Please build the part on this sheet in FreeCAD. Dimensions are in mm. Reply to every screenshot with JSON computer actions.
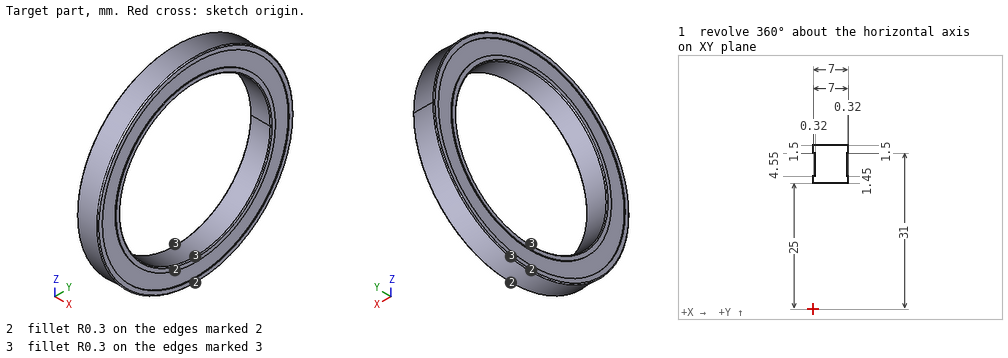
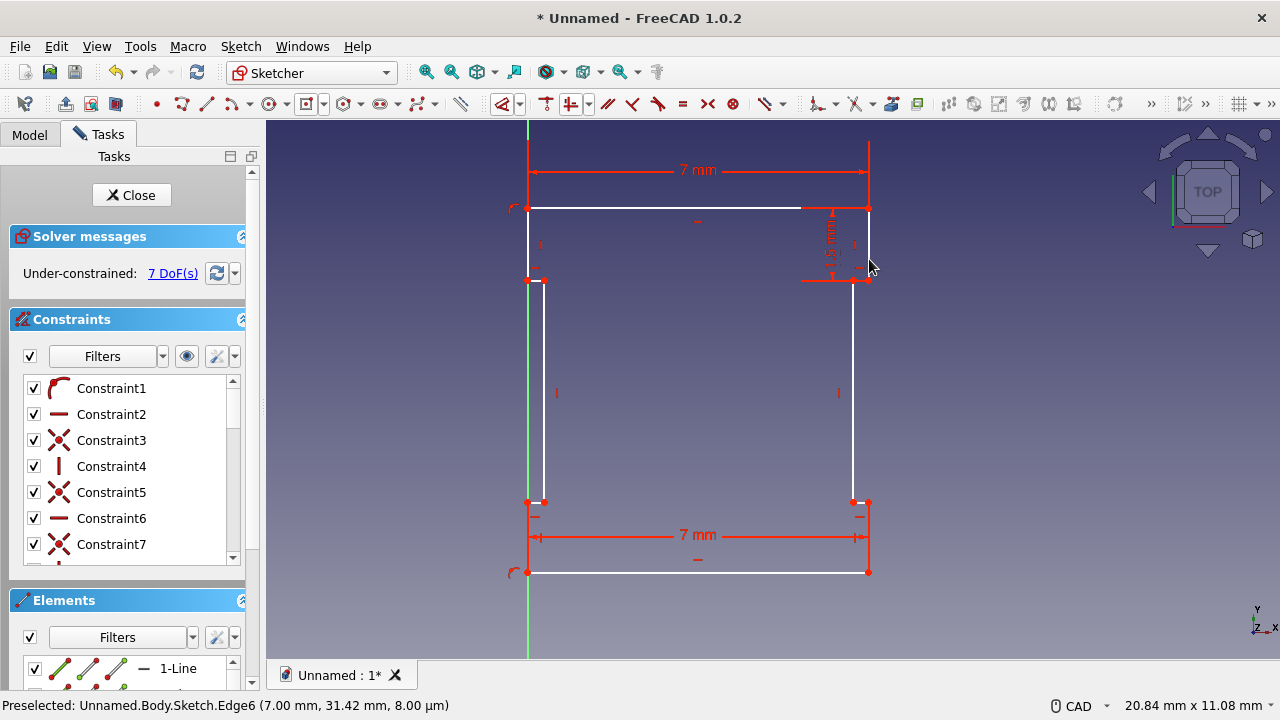
{"action": "left_click", "coordinate": [528, 230]}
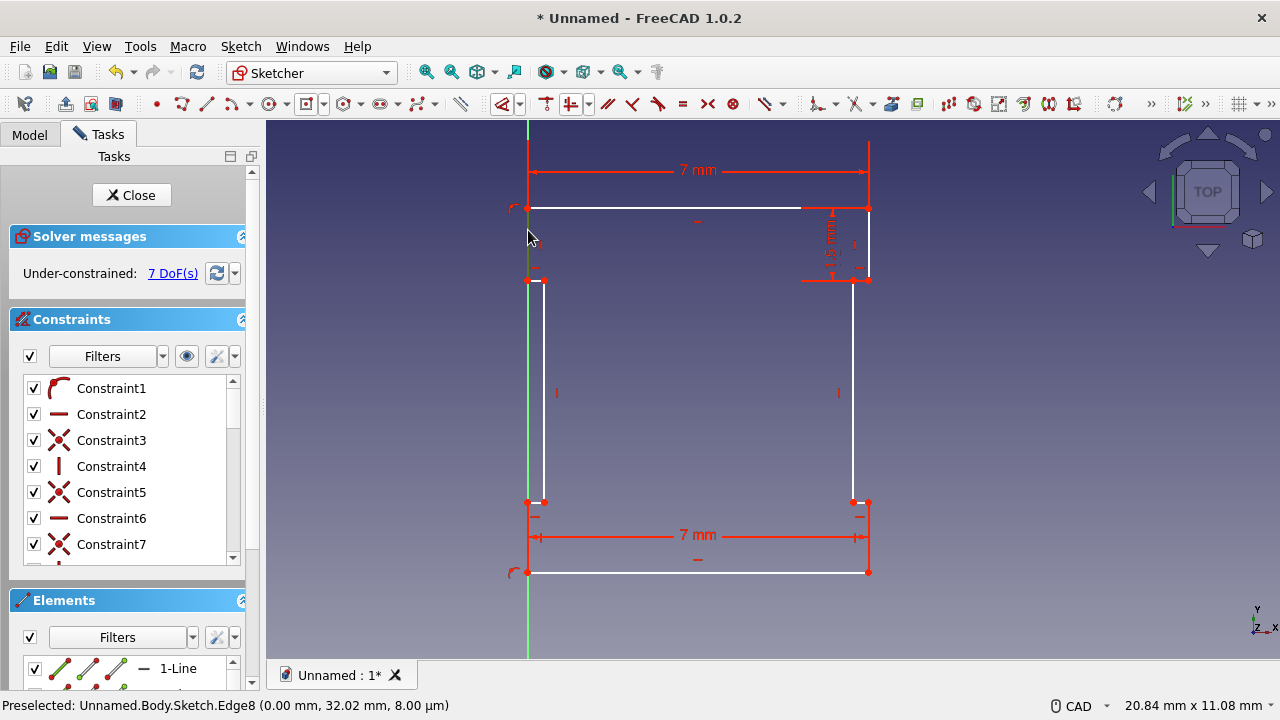
{"action": "left_click", "coordinate": [520, 104]}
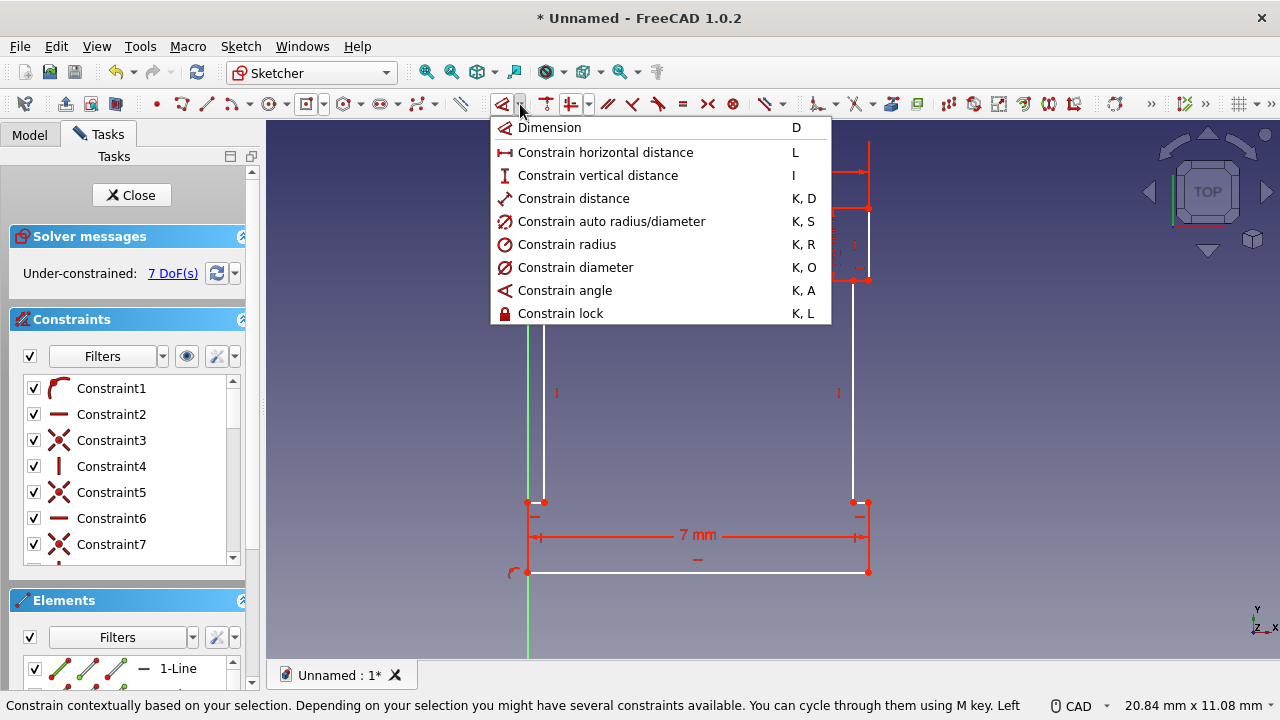
{"action": "left_click", "coordinate": [661, 176]}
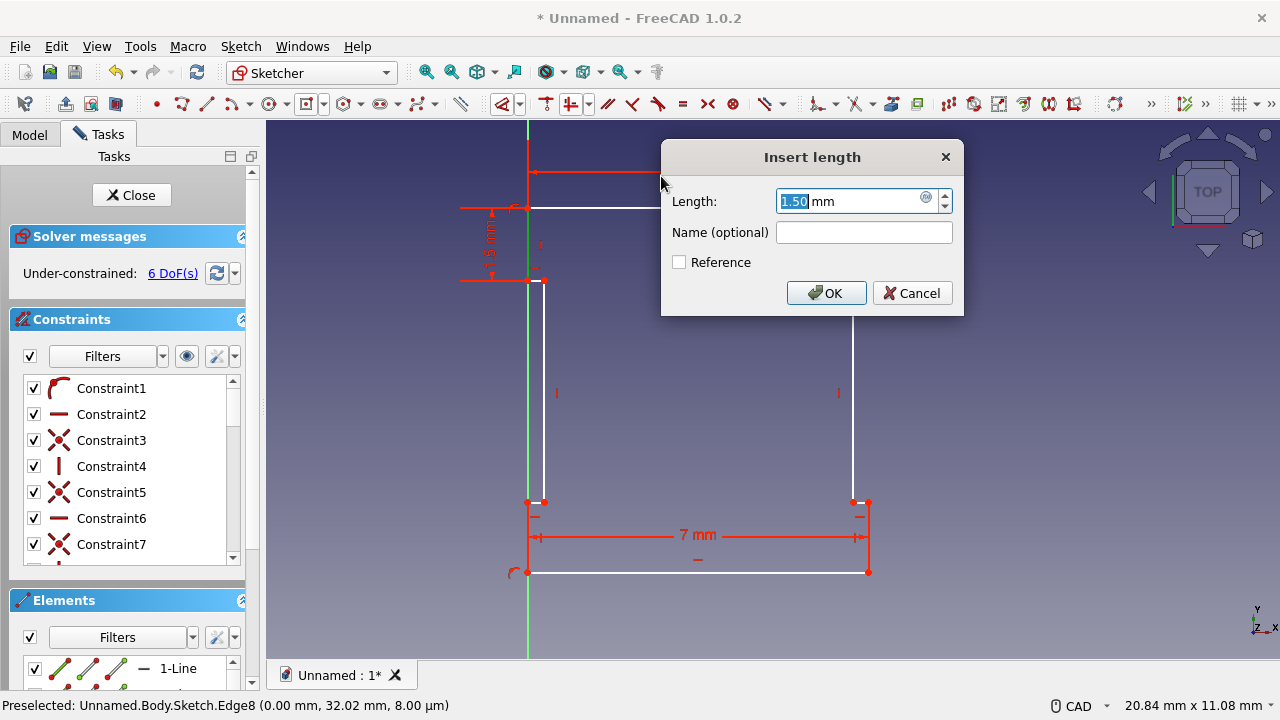
{"action": "type", "text": "1.5"}
{"action": "key", "text": "Return"}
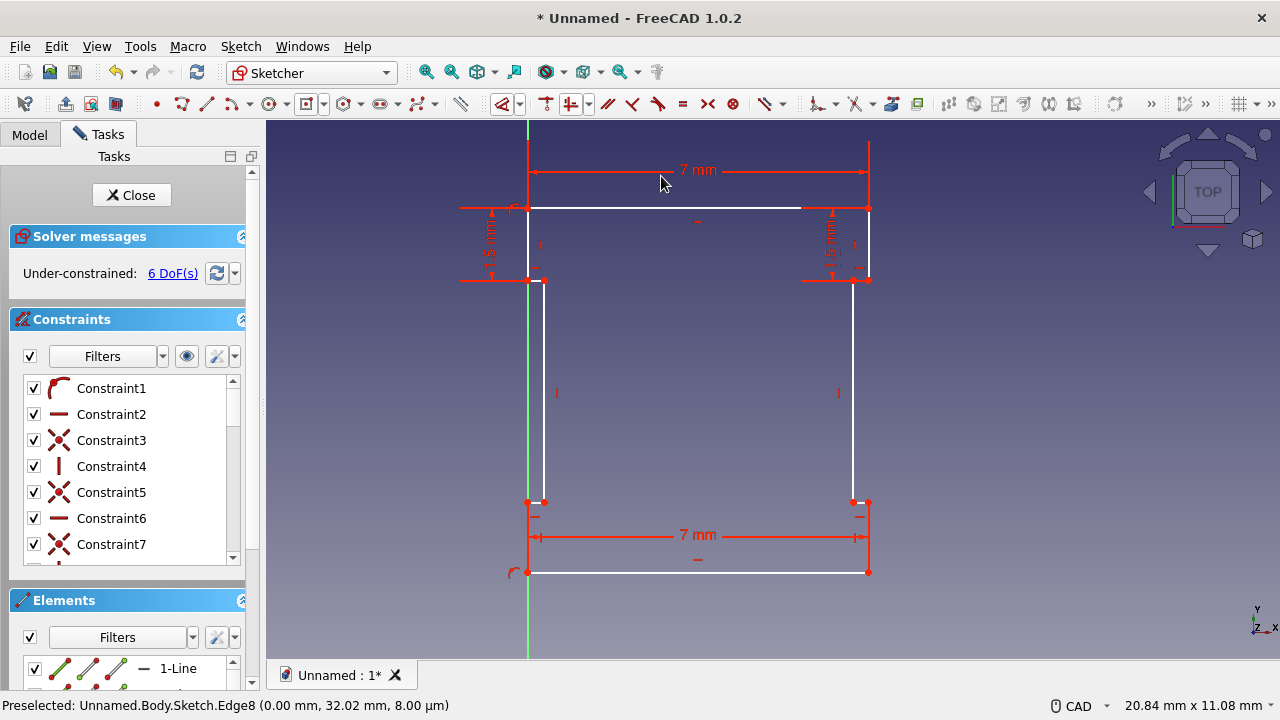
{"action": "left_click", "coordinate": [528, 573]}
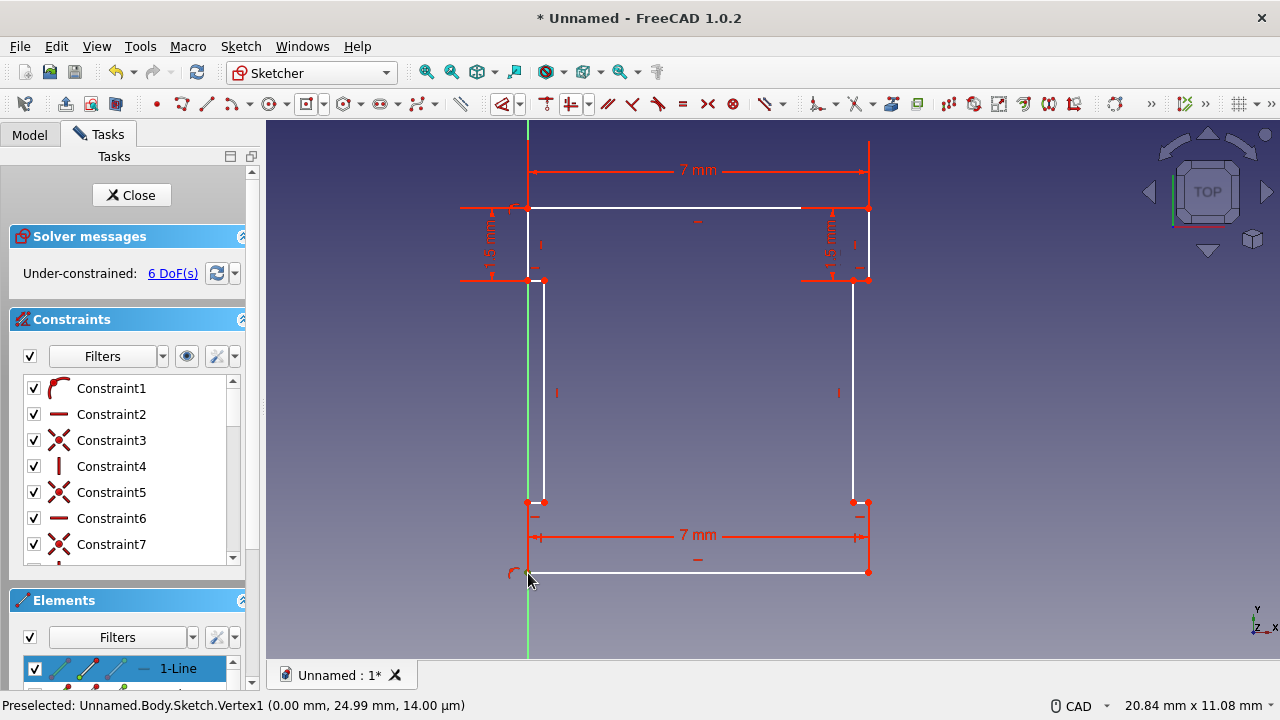
{"action": "key", "text": "i"}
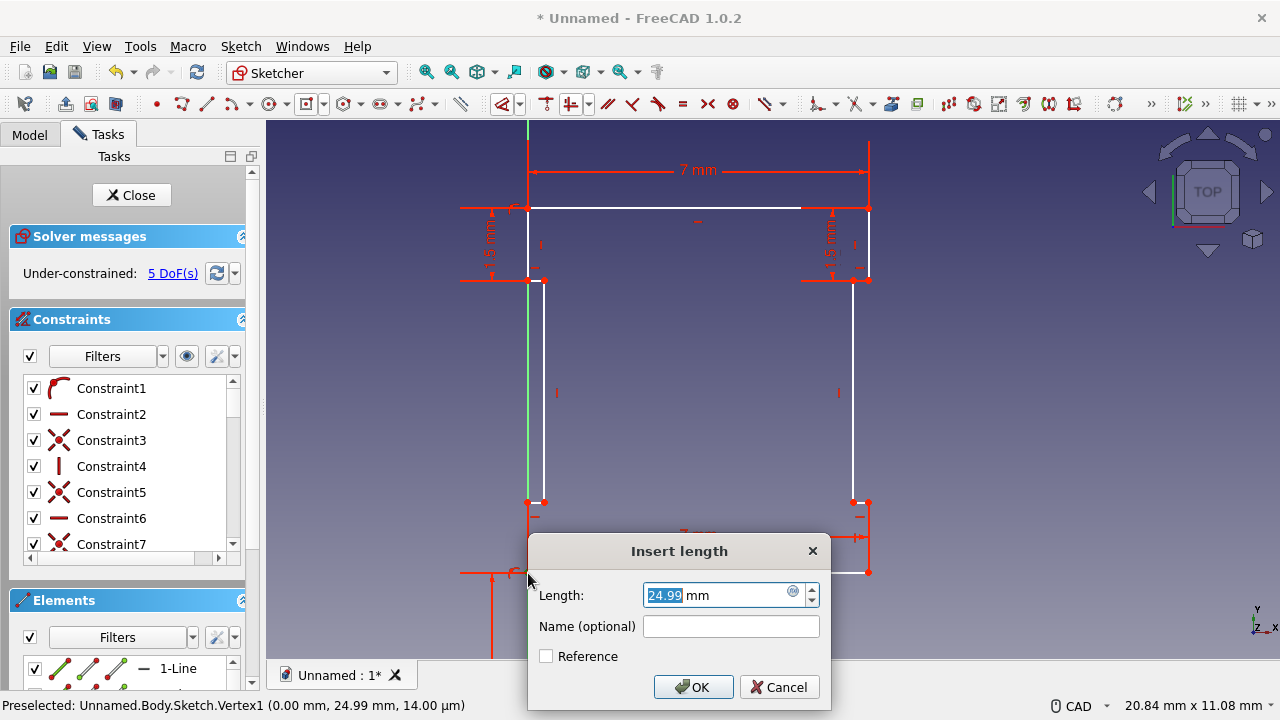
{"action": "type", "text": "25"}
{"action": "key", "text": "Return"}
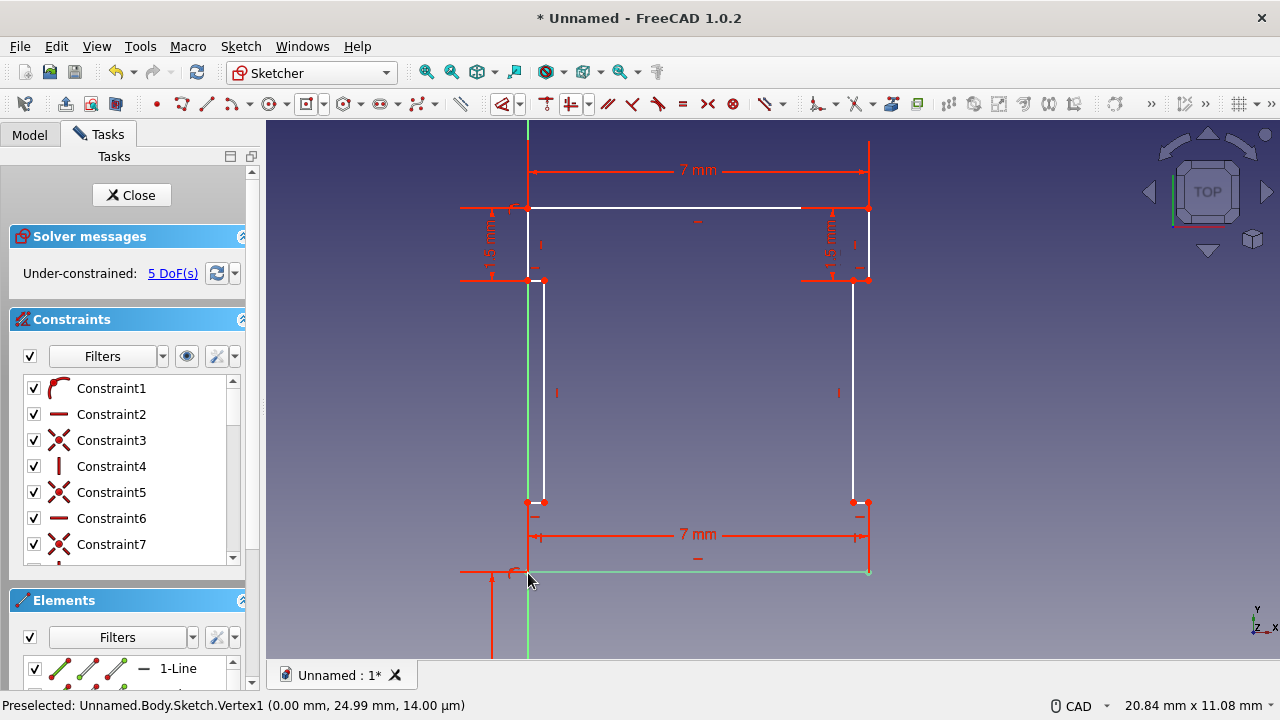
{"action": "left_click", "coordinate": [853, 281]}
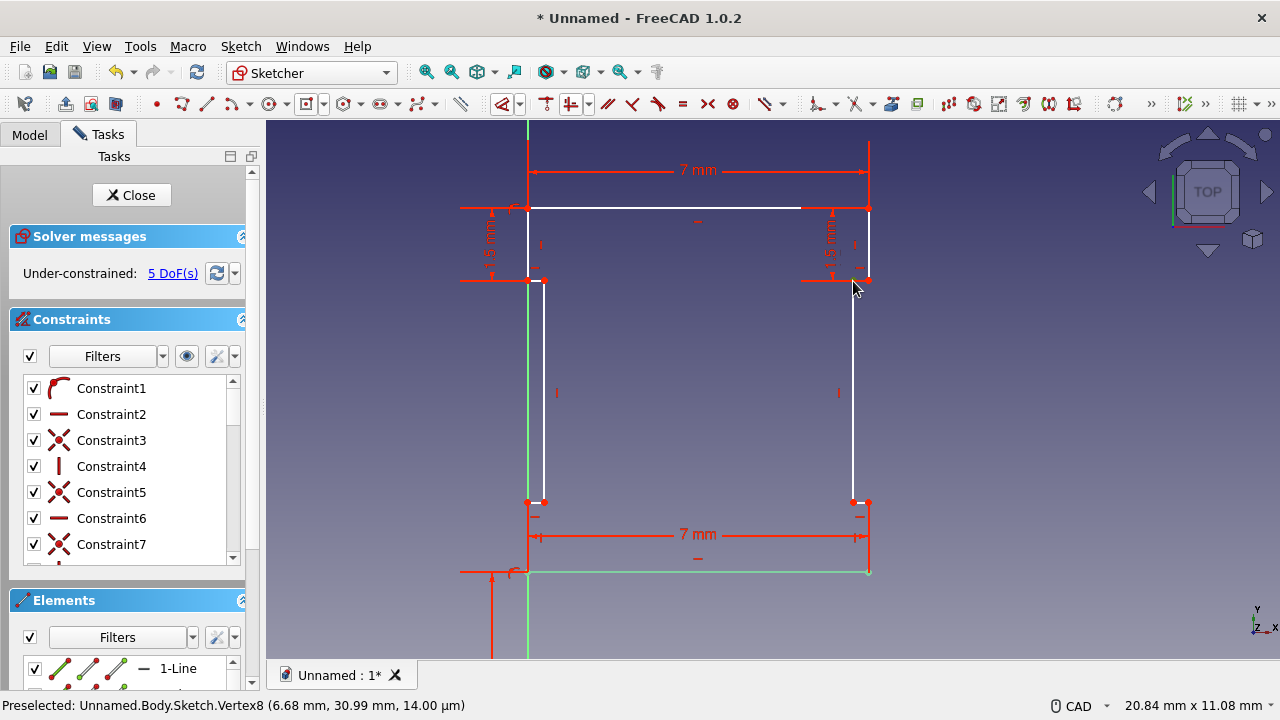
{"action": "key", "text": "i"}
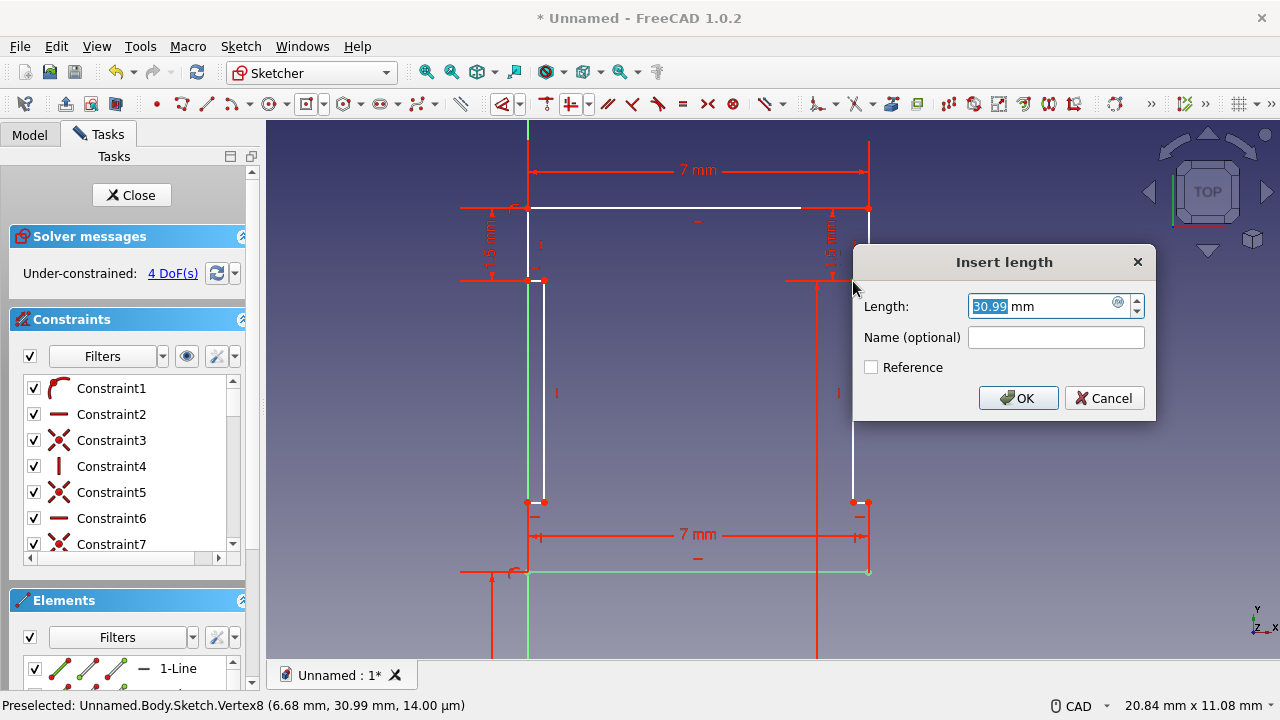
{"action": "type", "text": "31"}
{"action": "key", "text": "Return"}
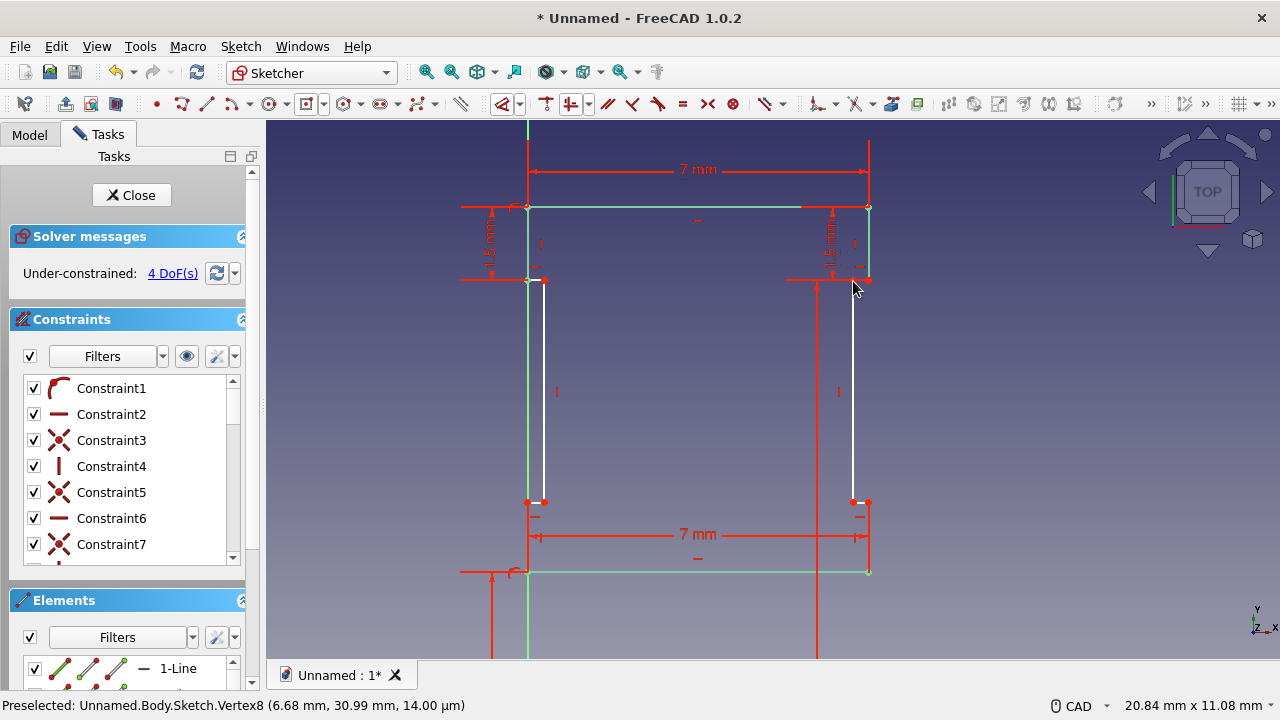
{"action": "left_click", "coordinate": [869, 552]}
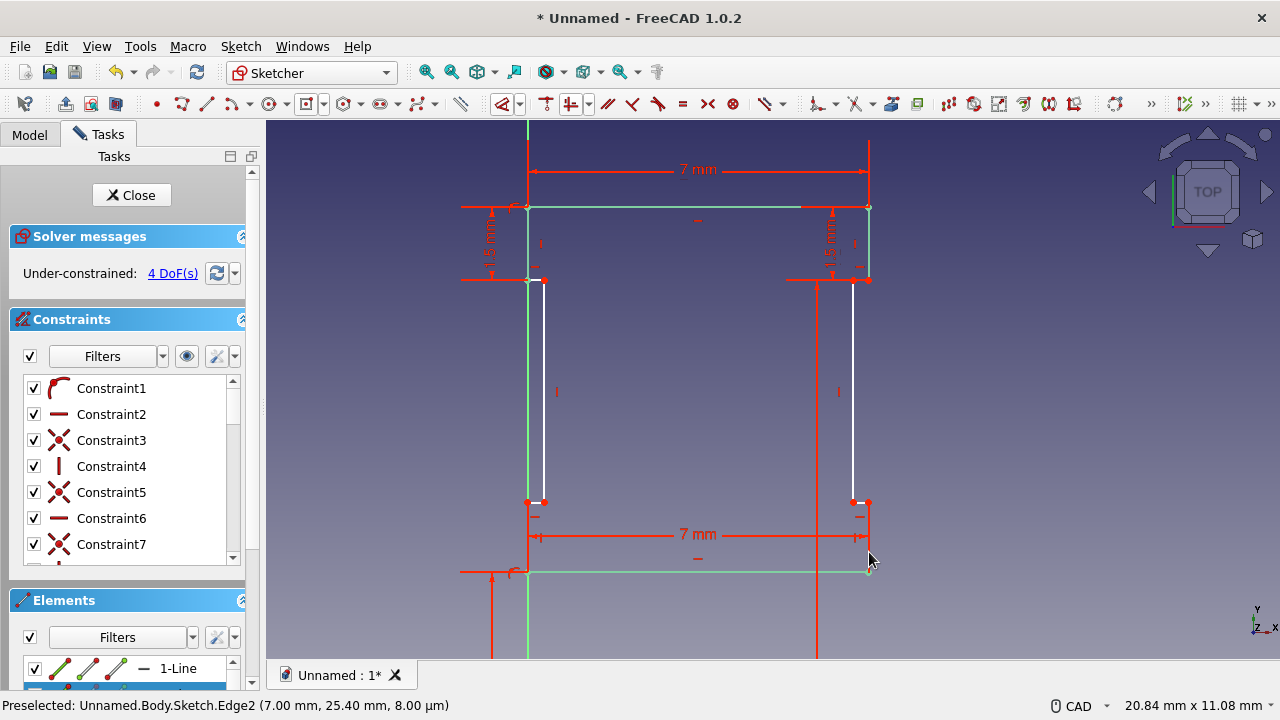
{"action": "left_click", "coordinate": [520, 104]}